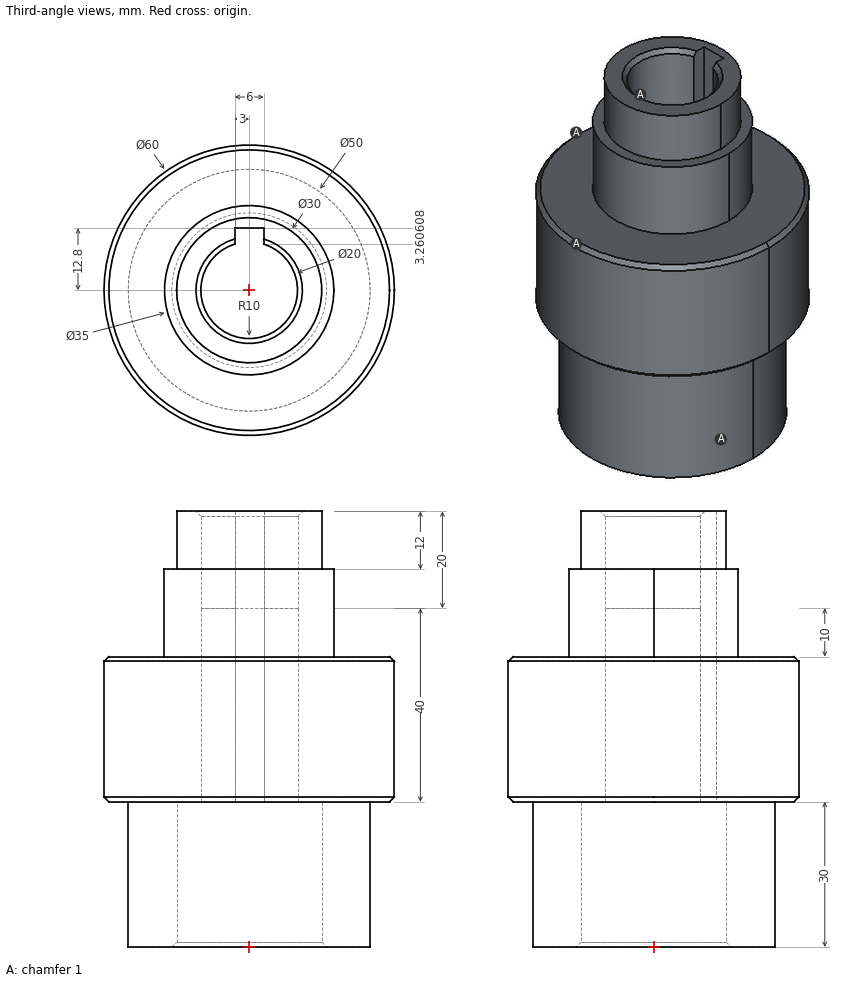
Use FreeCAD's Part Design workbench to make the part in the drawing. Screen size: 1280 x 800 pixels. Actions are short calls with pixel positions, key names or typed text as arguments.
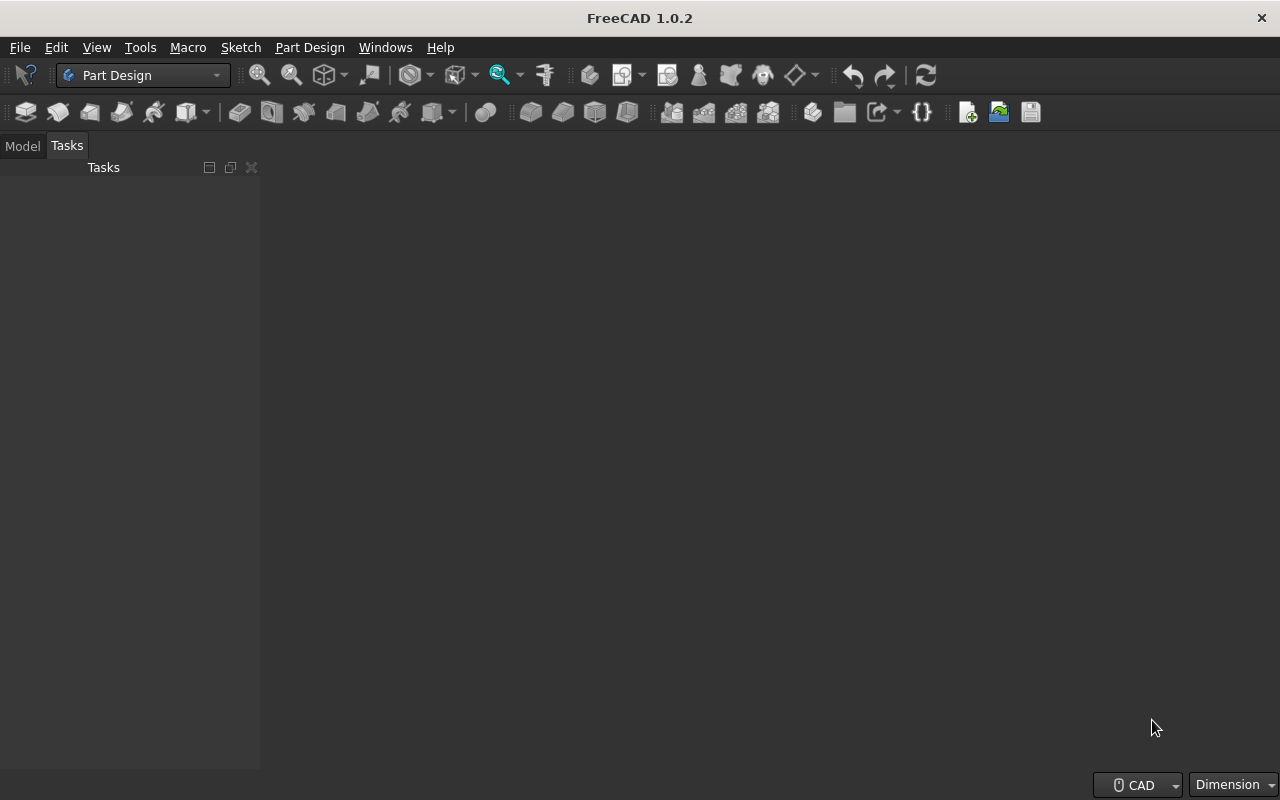
click(968, 112)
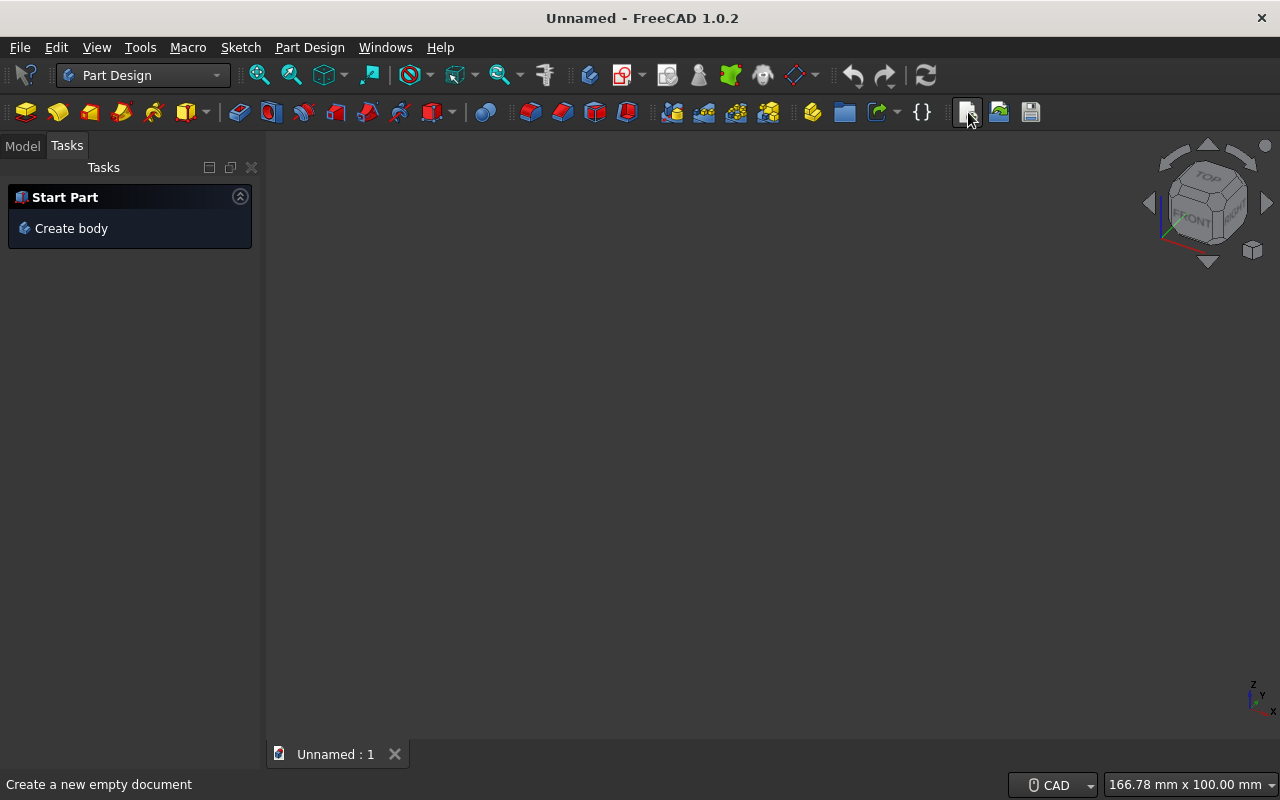
click(622, 76)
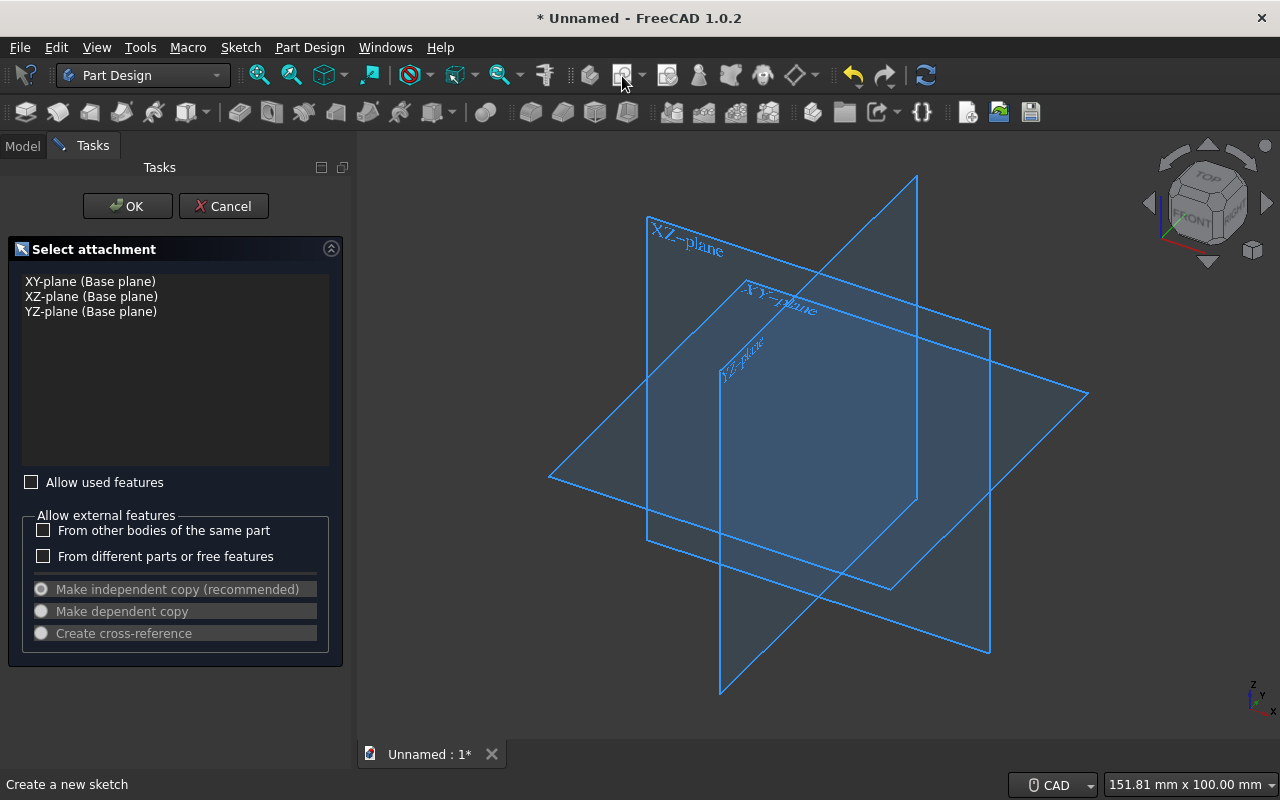
click(82, 282)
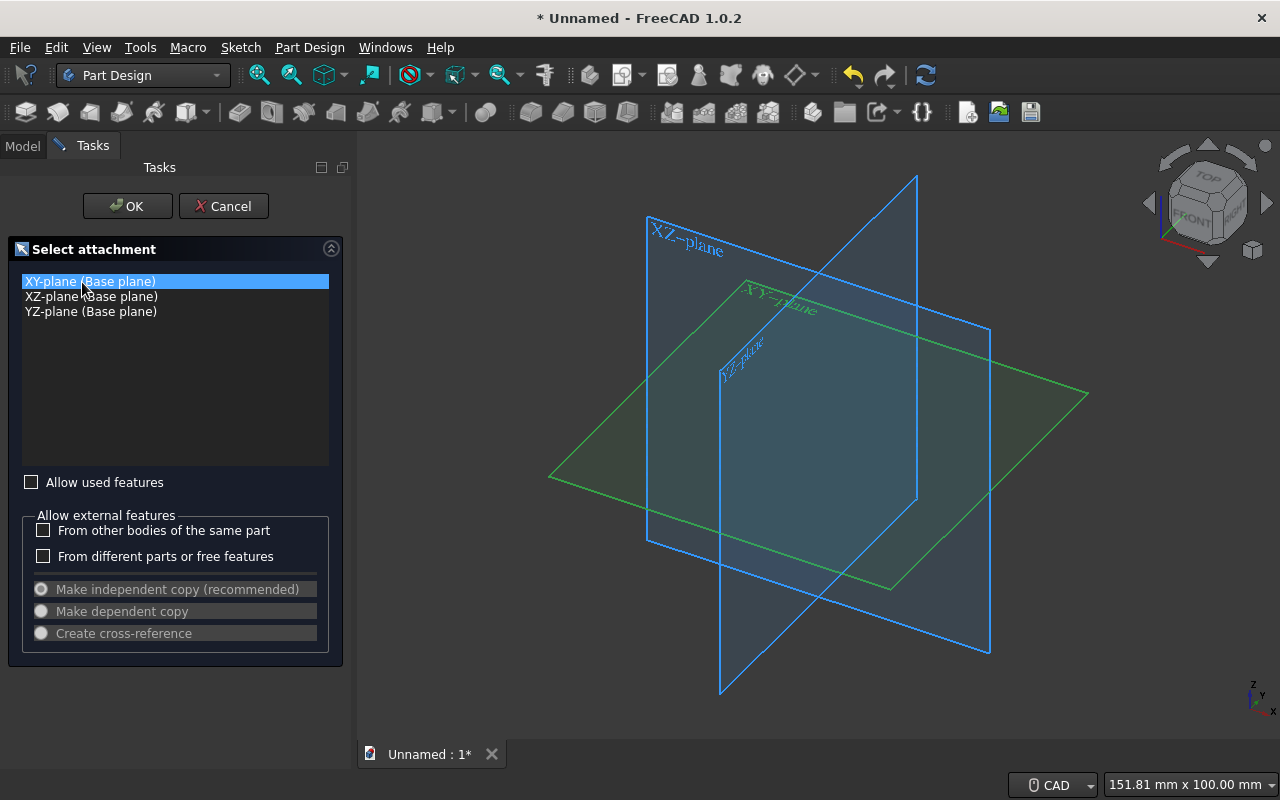
click(128, 206)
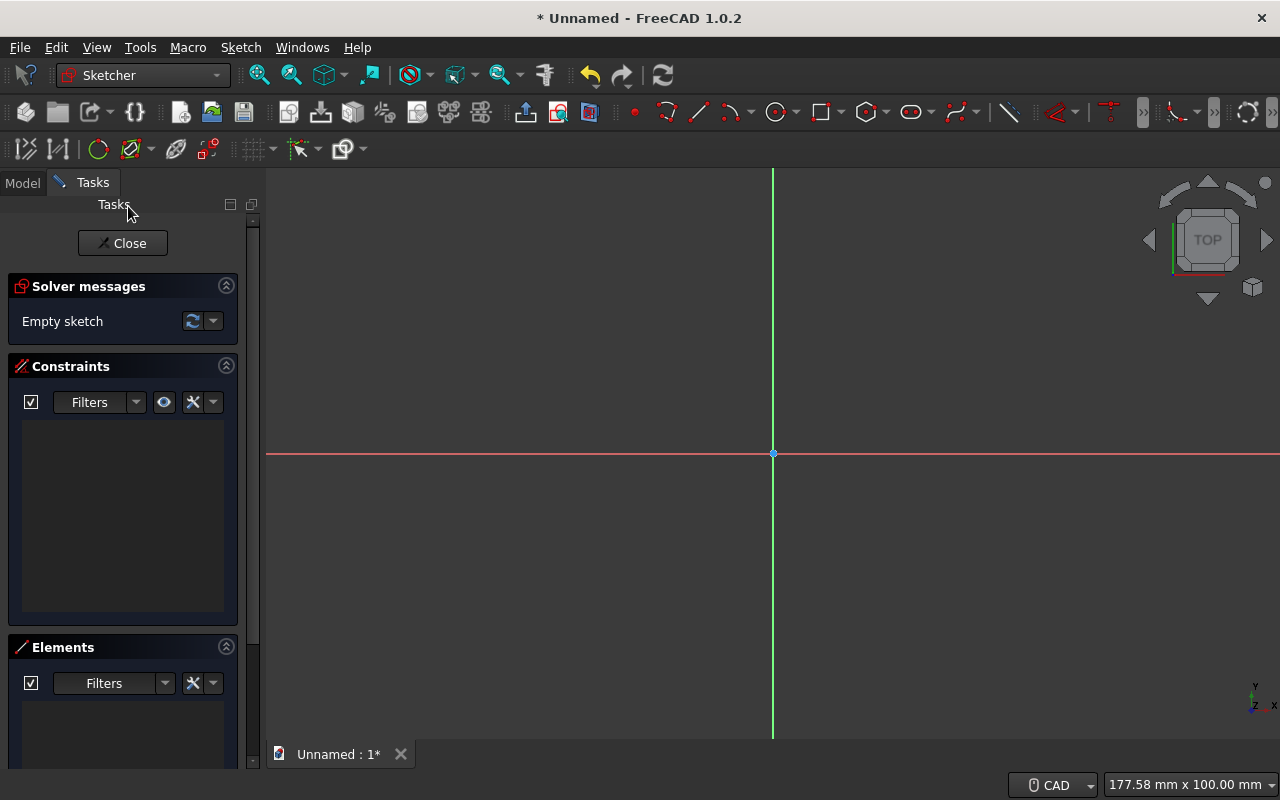
click(776, 112)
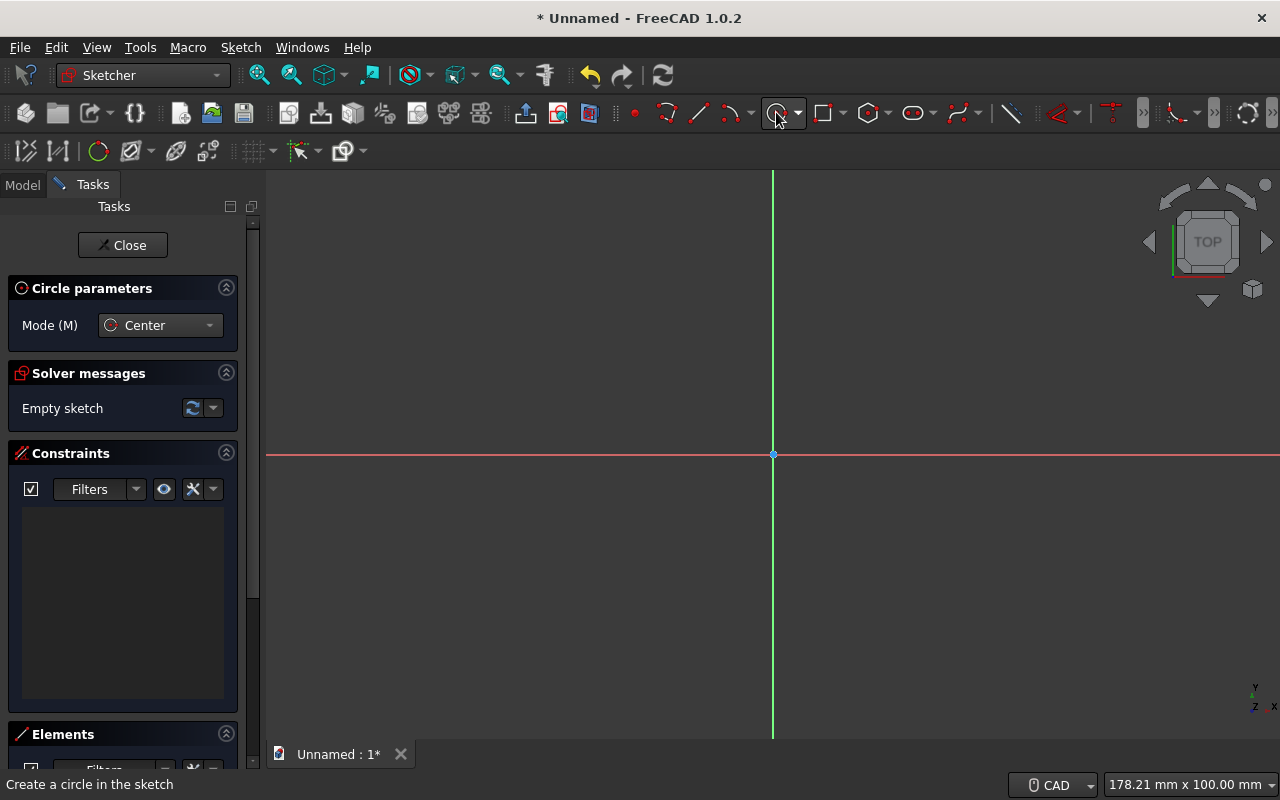
click(773, 454)
move(874, 354)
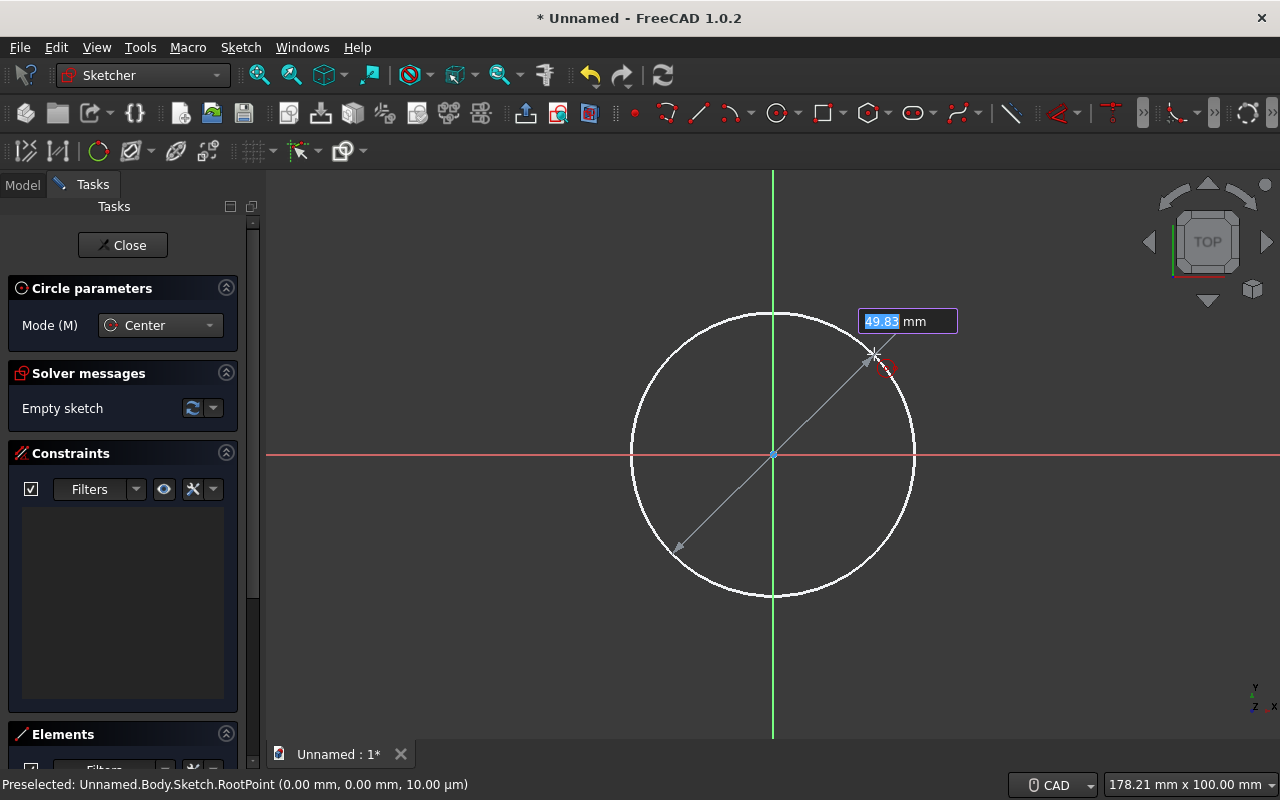
text(50)
key(Return)
key(Escape)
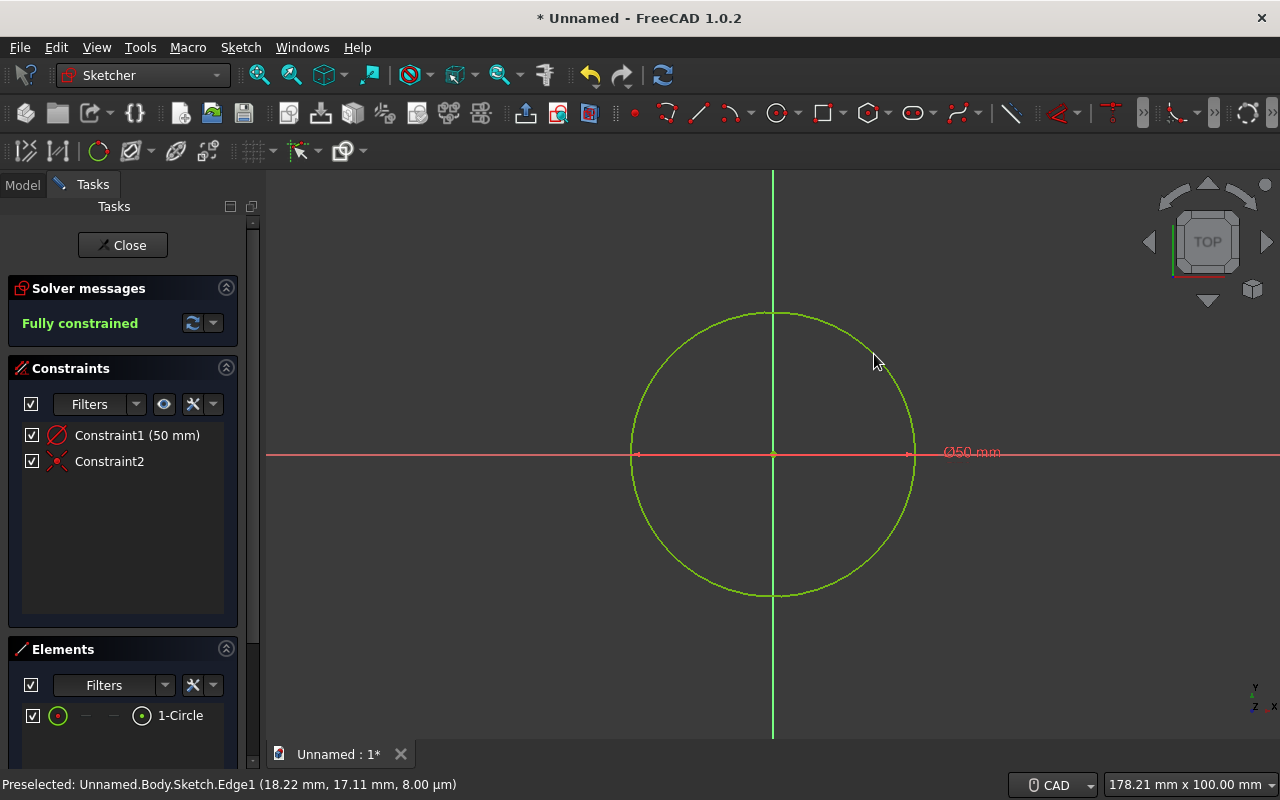
click(123, 245)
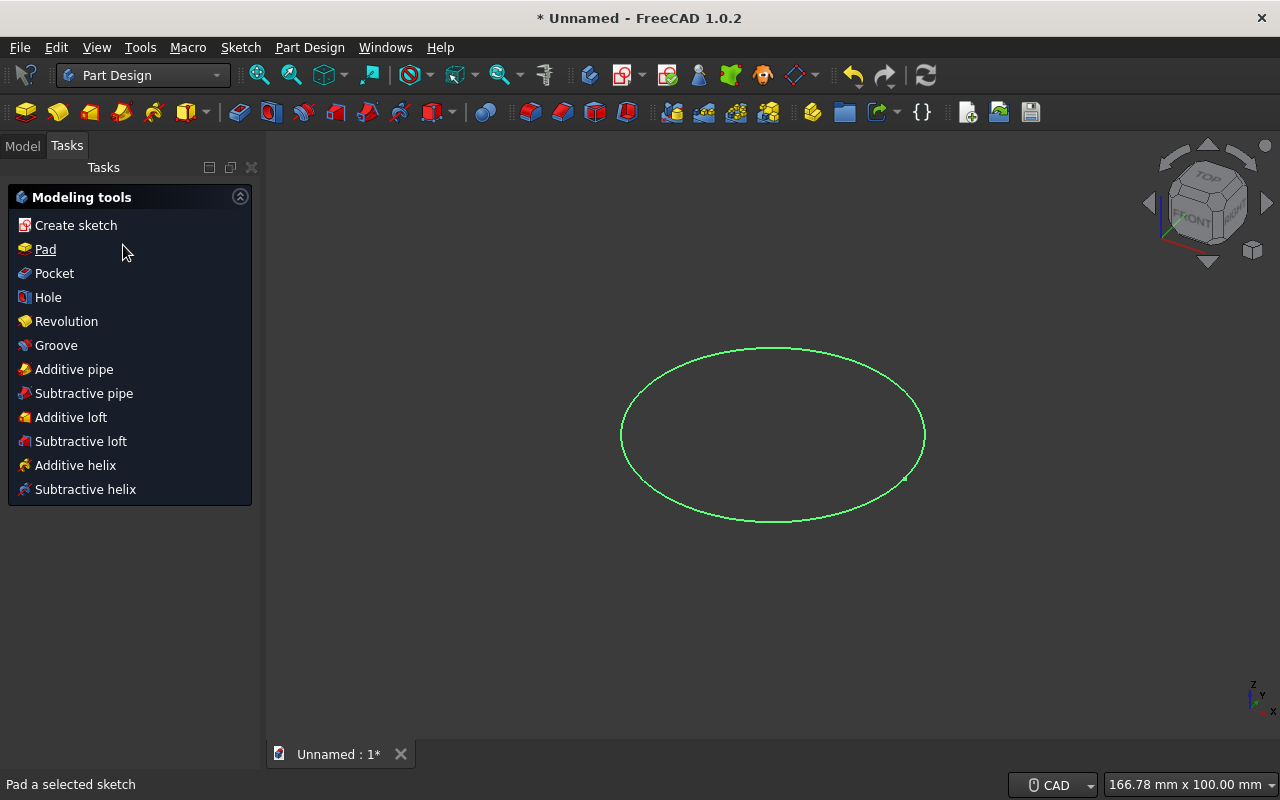
click(26, 112)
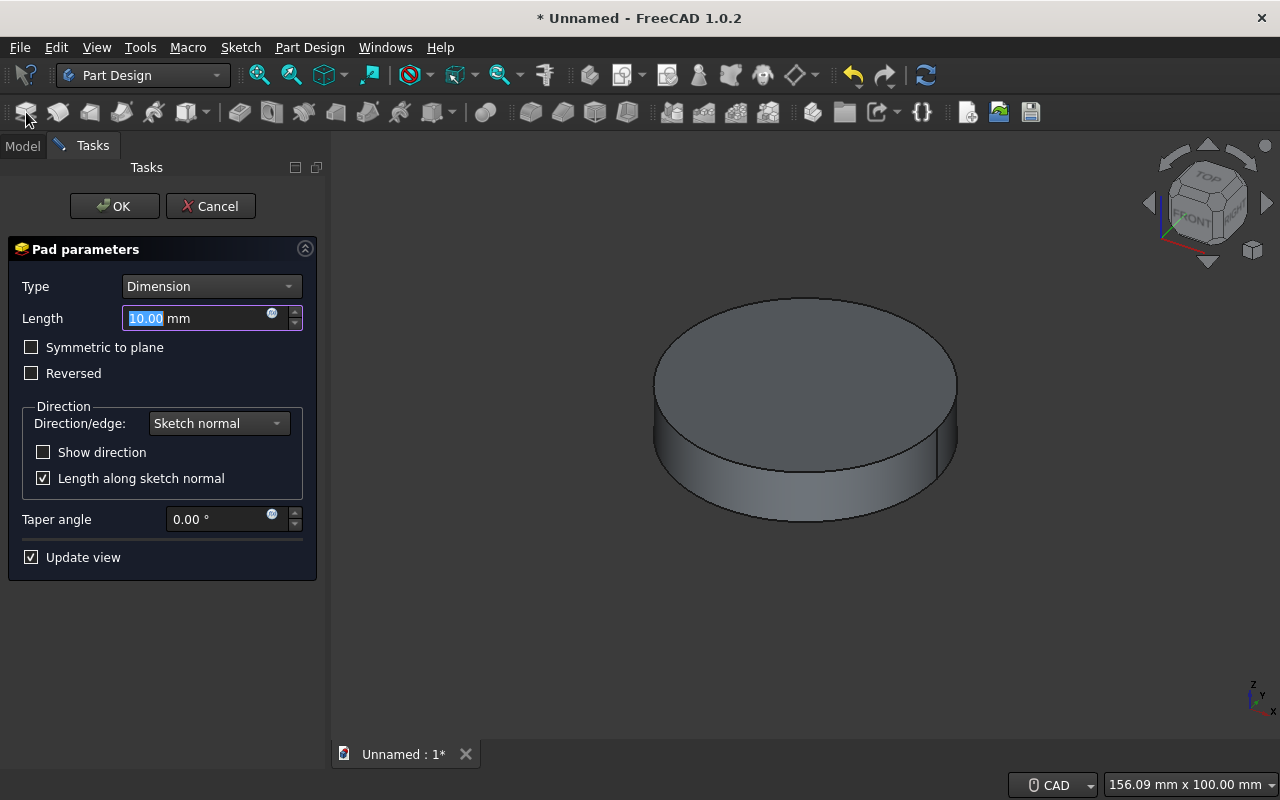
text(30)
key(Tab)